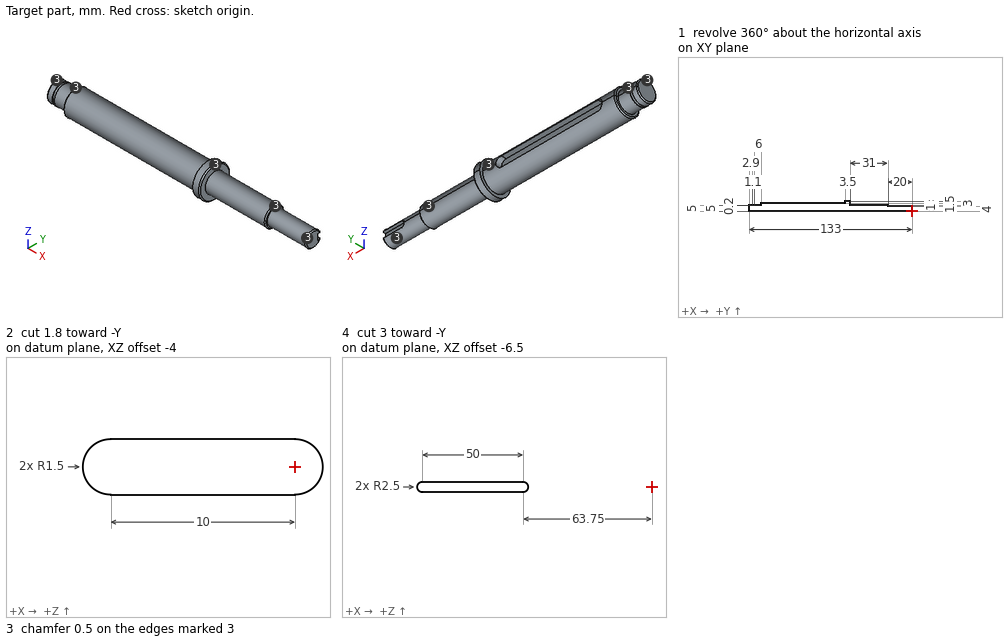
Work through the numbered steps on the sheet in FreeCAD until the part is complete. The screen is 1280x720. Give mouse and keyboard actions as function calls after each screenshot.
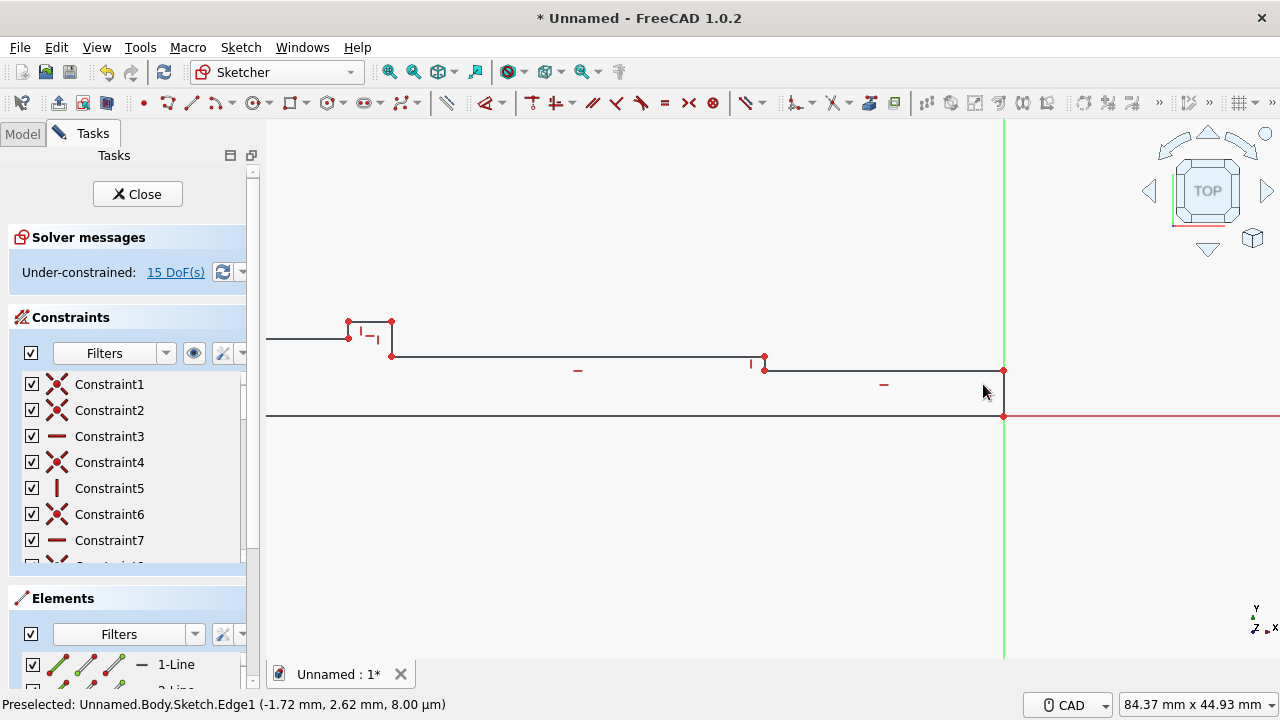
scroll(995, 401, down, 5)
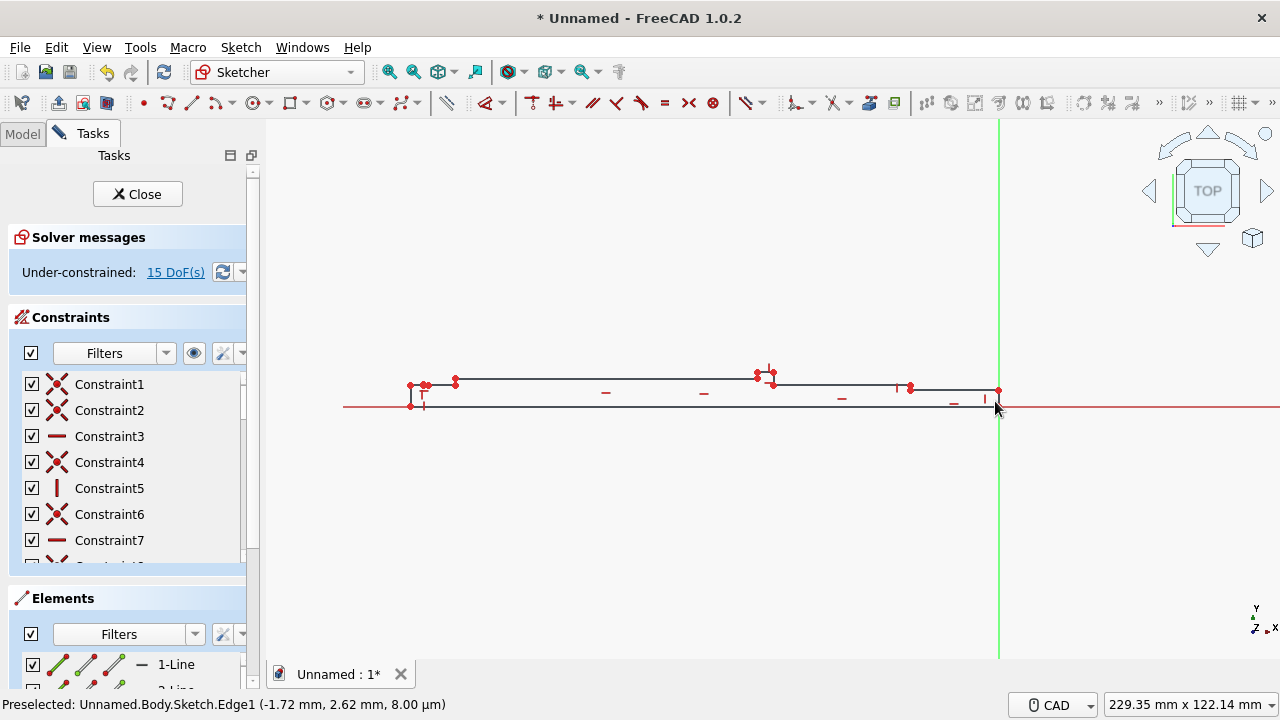
scroll(420, 385, up, 7)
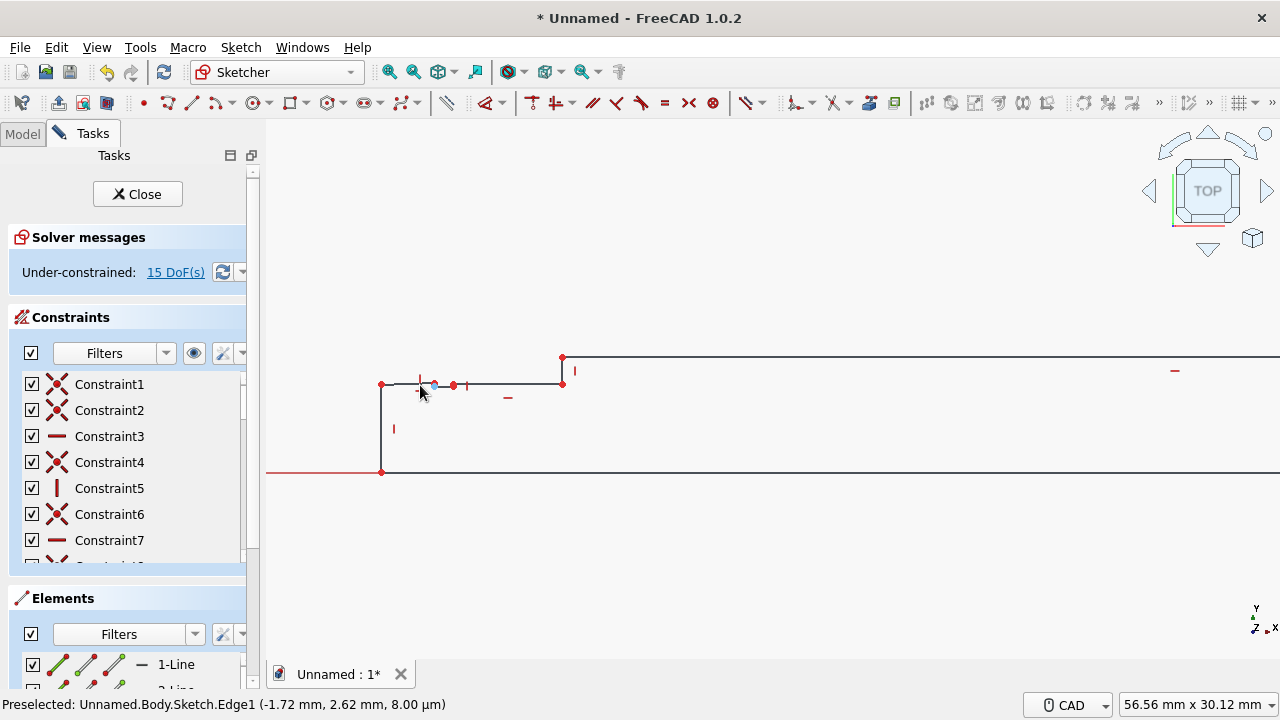
click(397, 384)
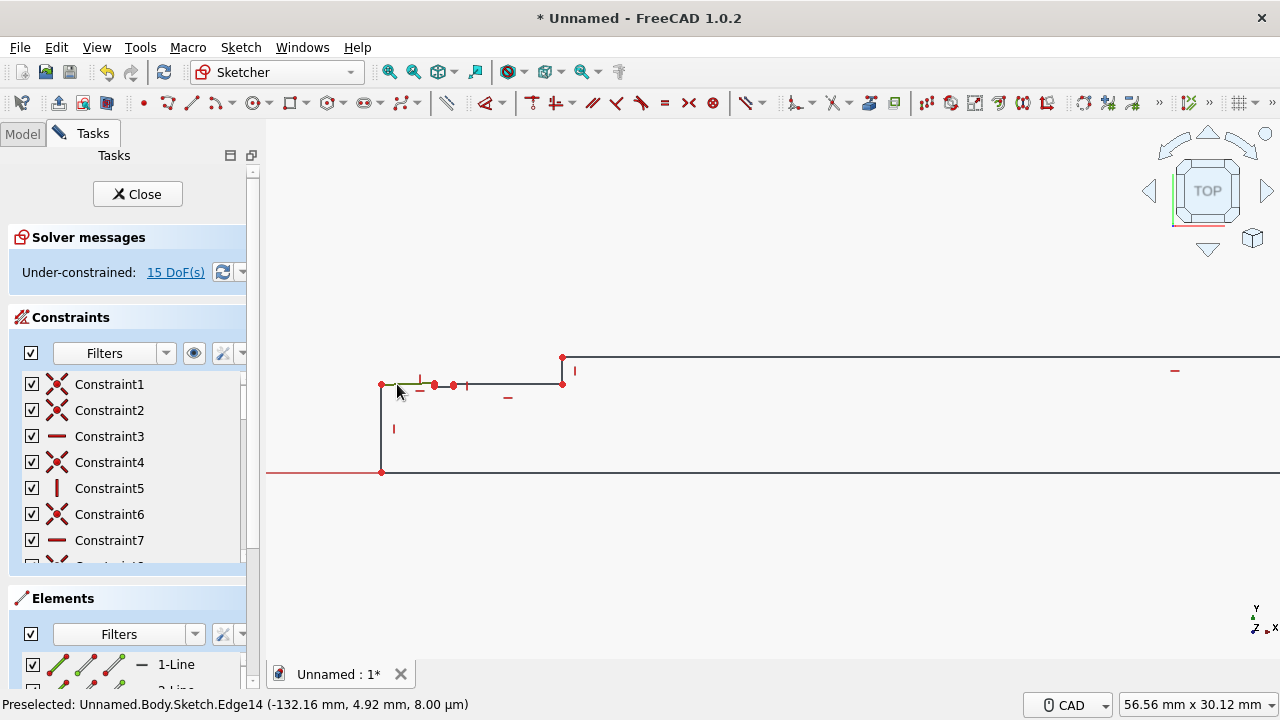
click(574, 104)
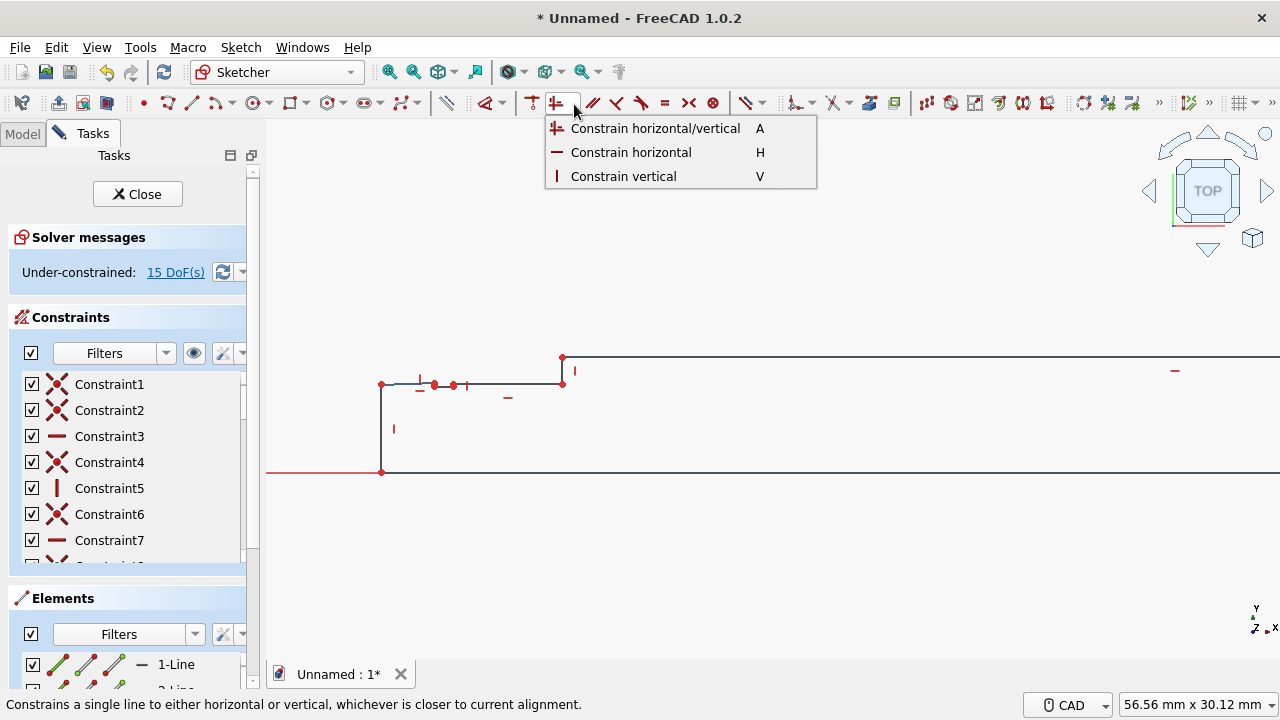
click(681, 152)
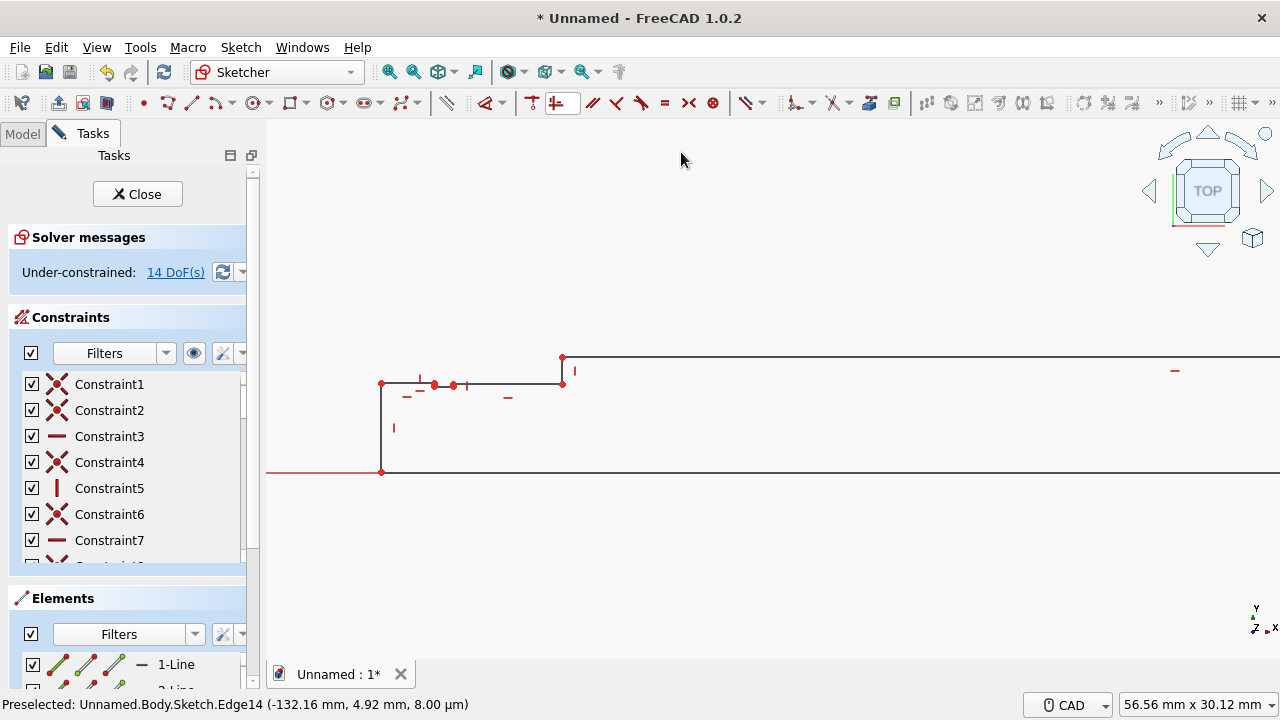
click(486, 104)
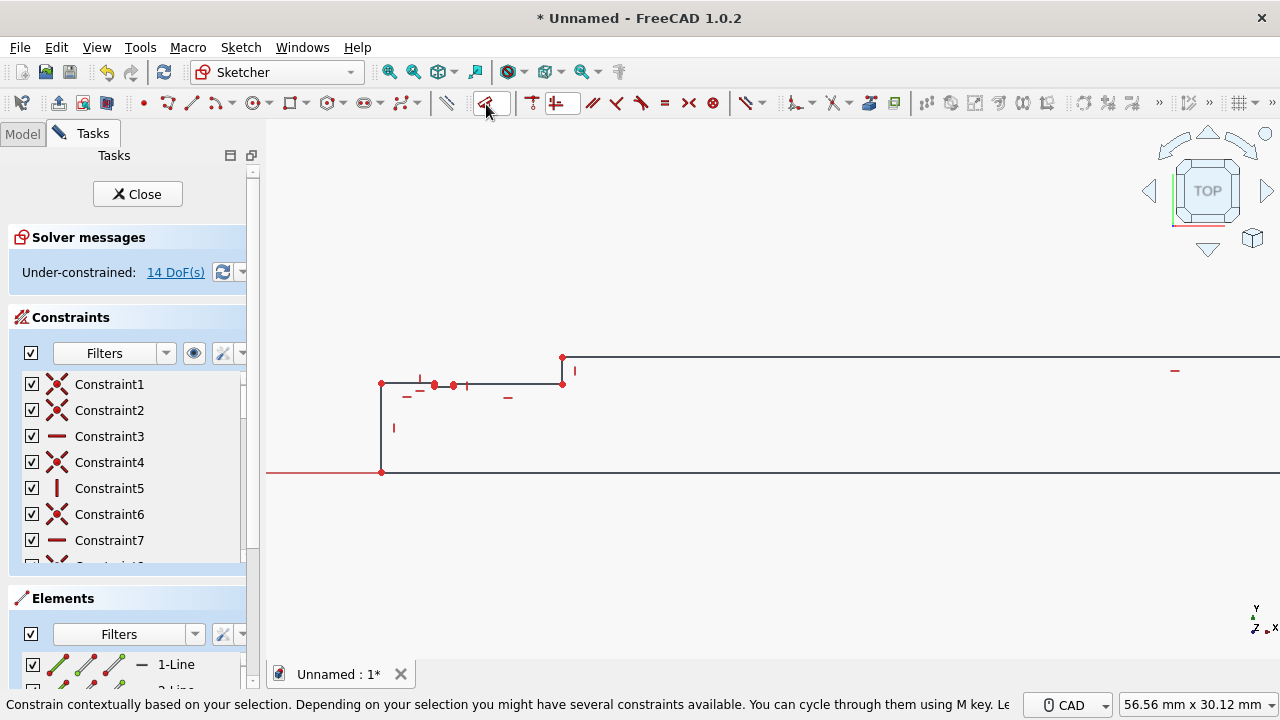
scroll(420, 385, down, 7)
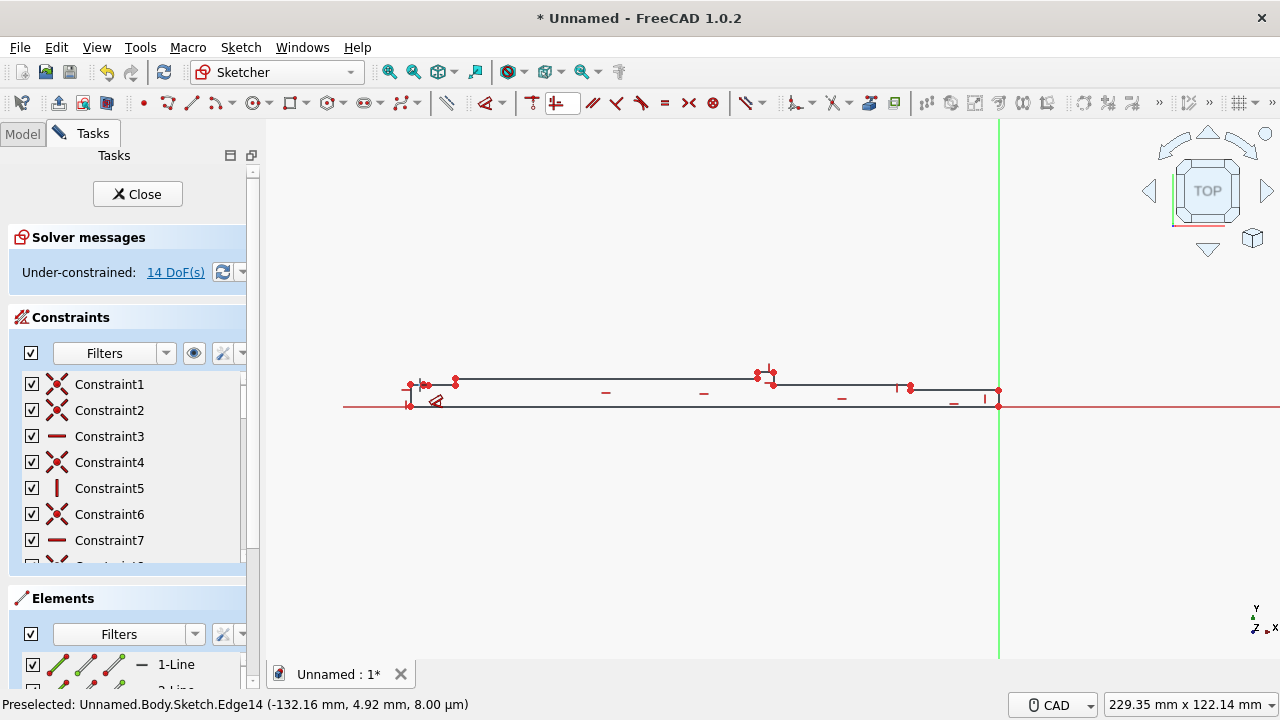
scroll(999, 402, up, 6)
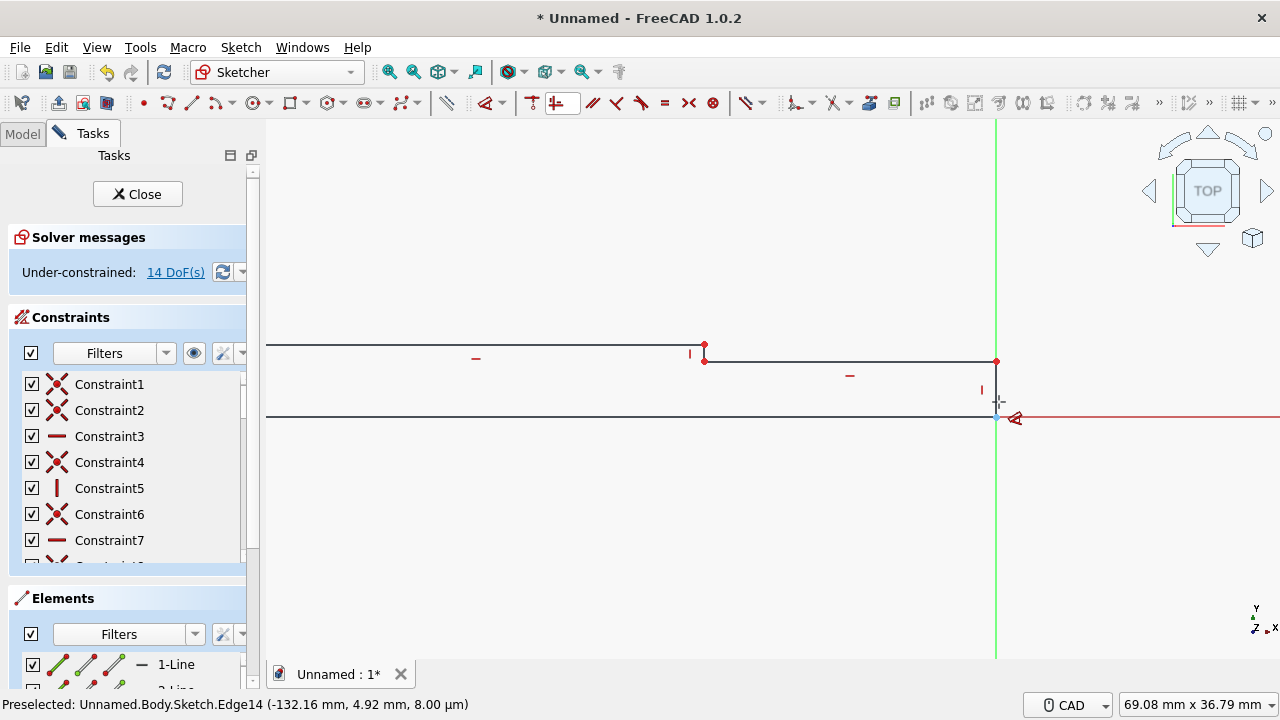
click(996, 401)
click(1030, 390)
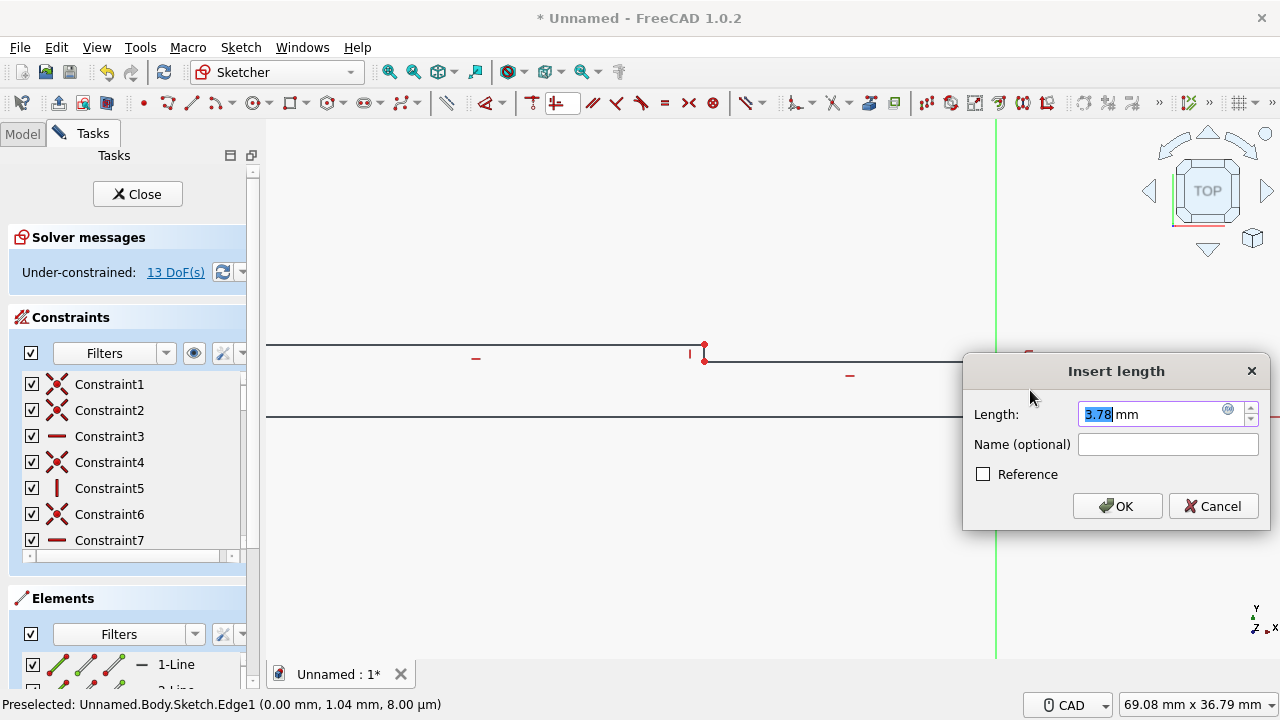
text(4)
key(Return)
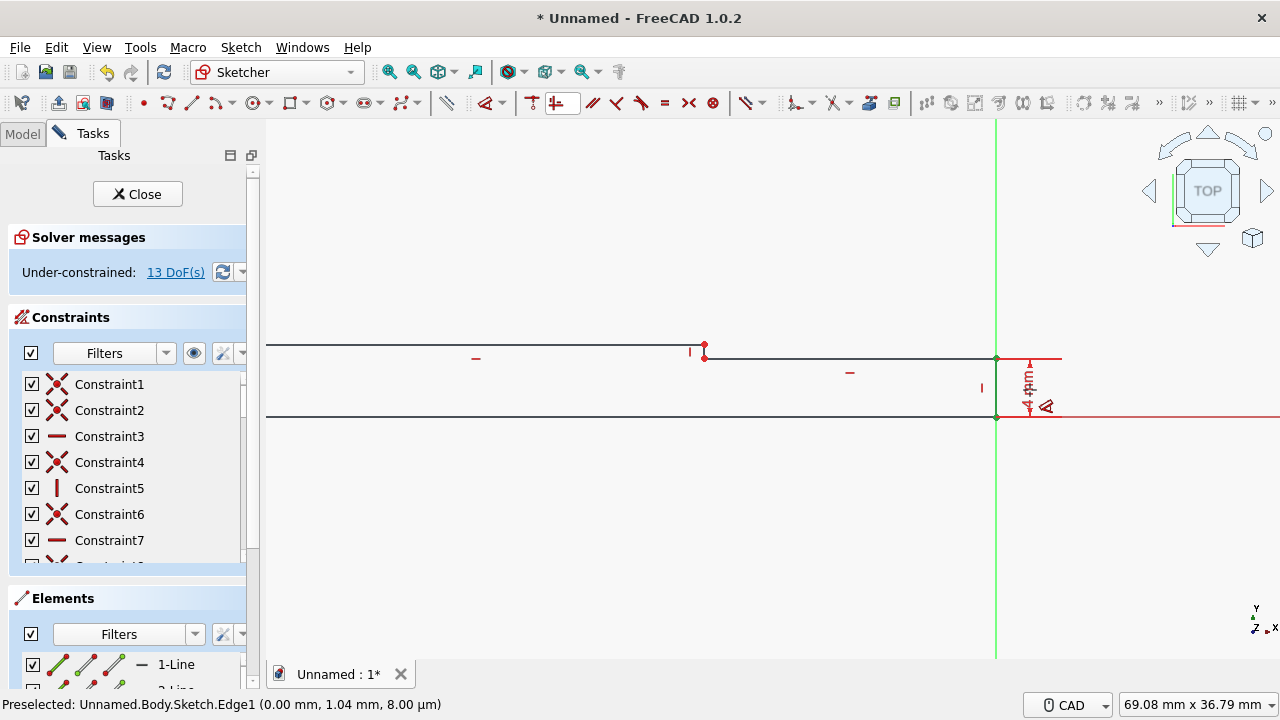
scroll(704, 352, up, 5)